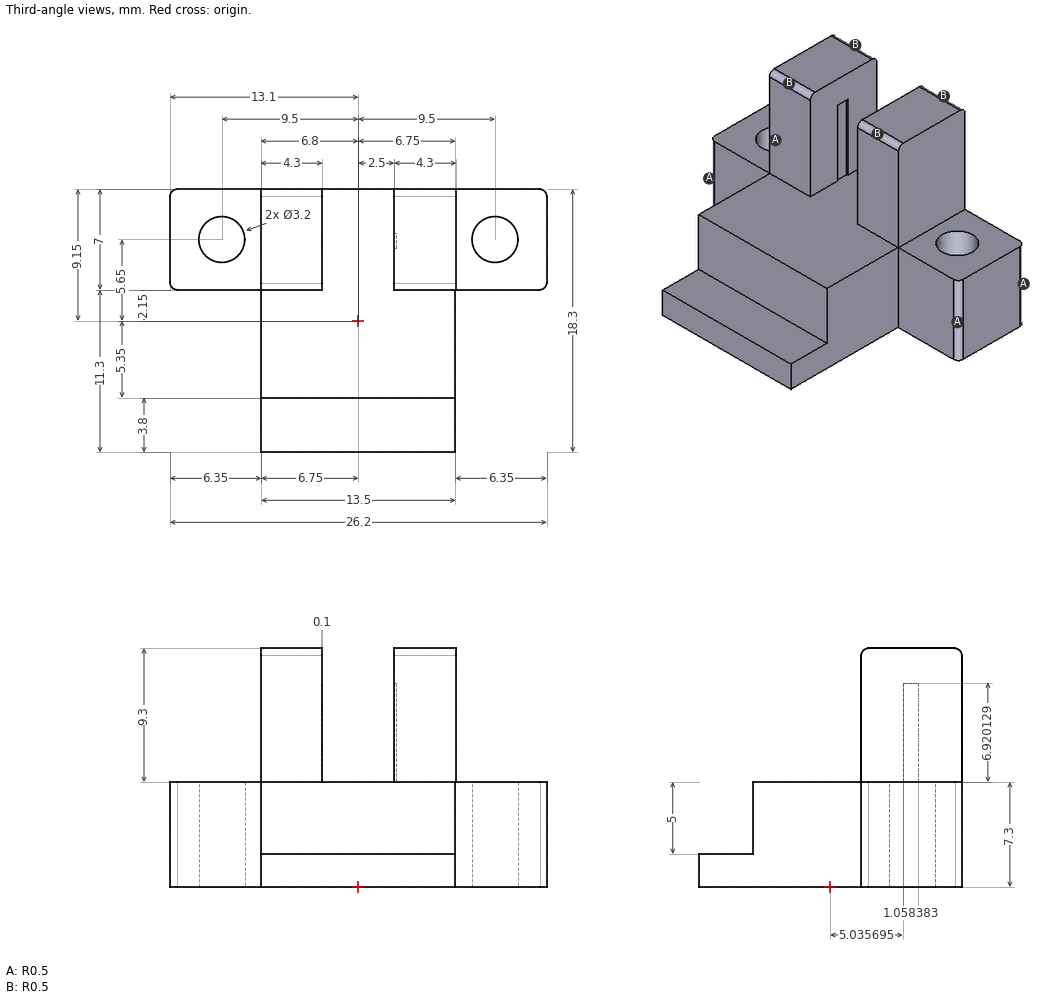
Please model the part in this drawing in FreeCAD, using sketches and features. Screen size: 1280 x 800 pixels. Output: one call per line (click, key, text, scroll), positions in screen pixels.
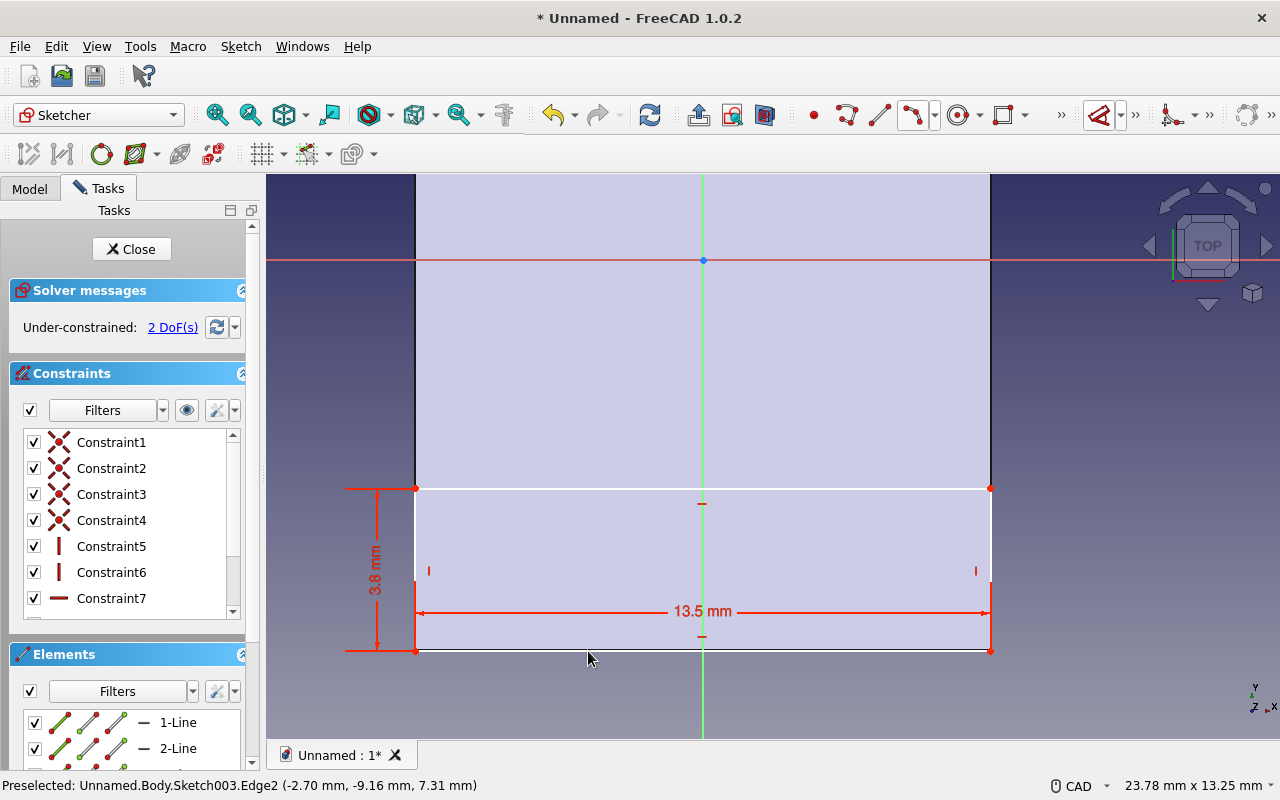
click(415, 489)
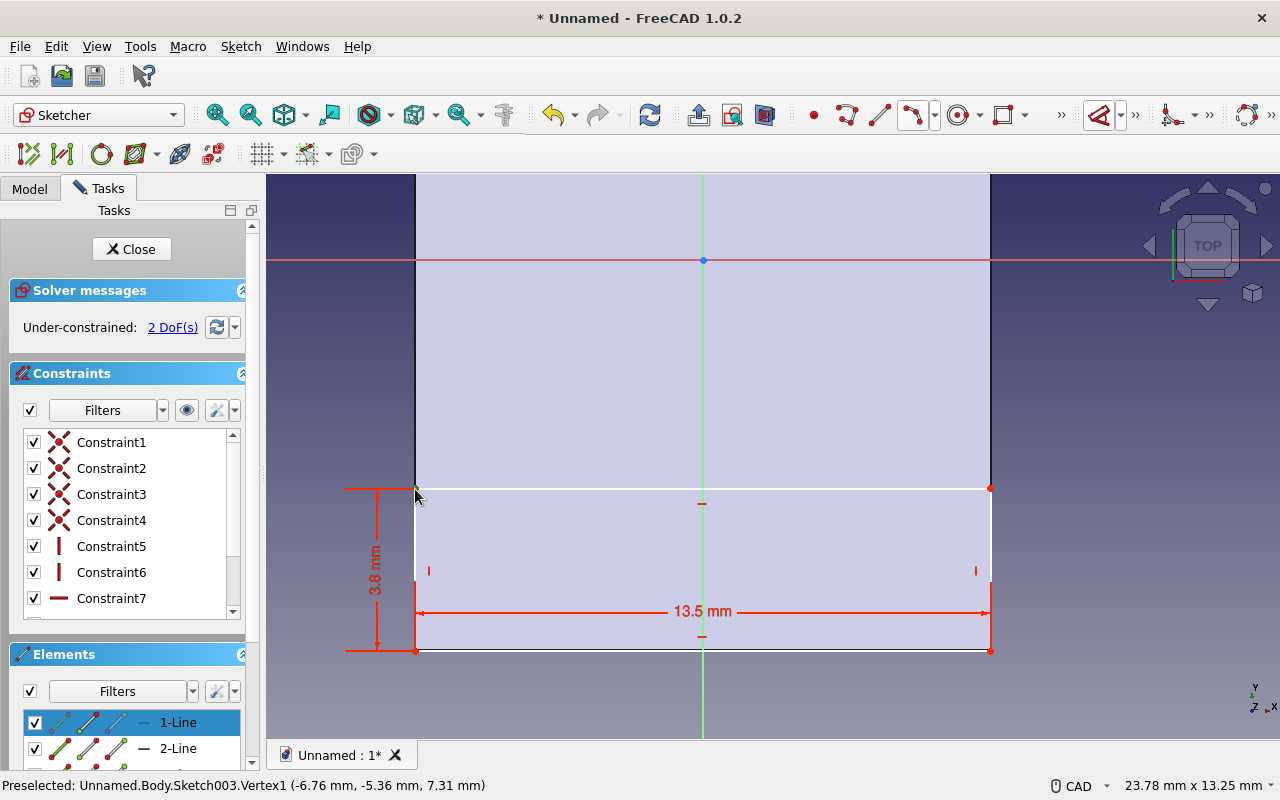
key(l)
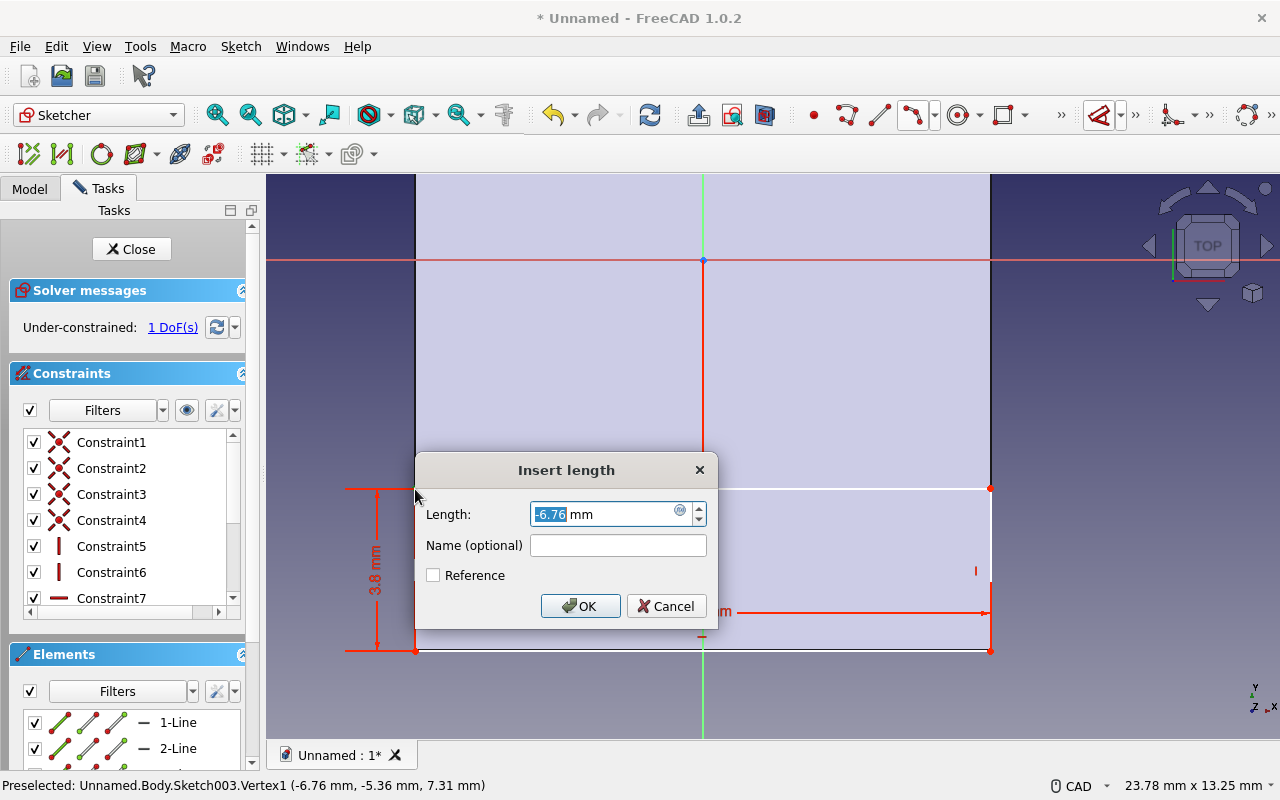
text(-6.75)
key(Return)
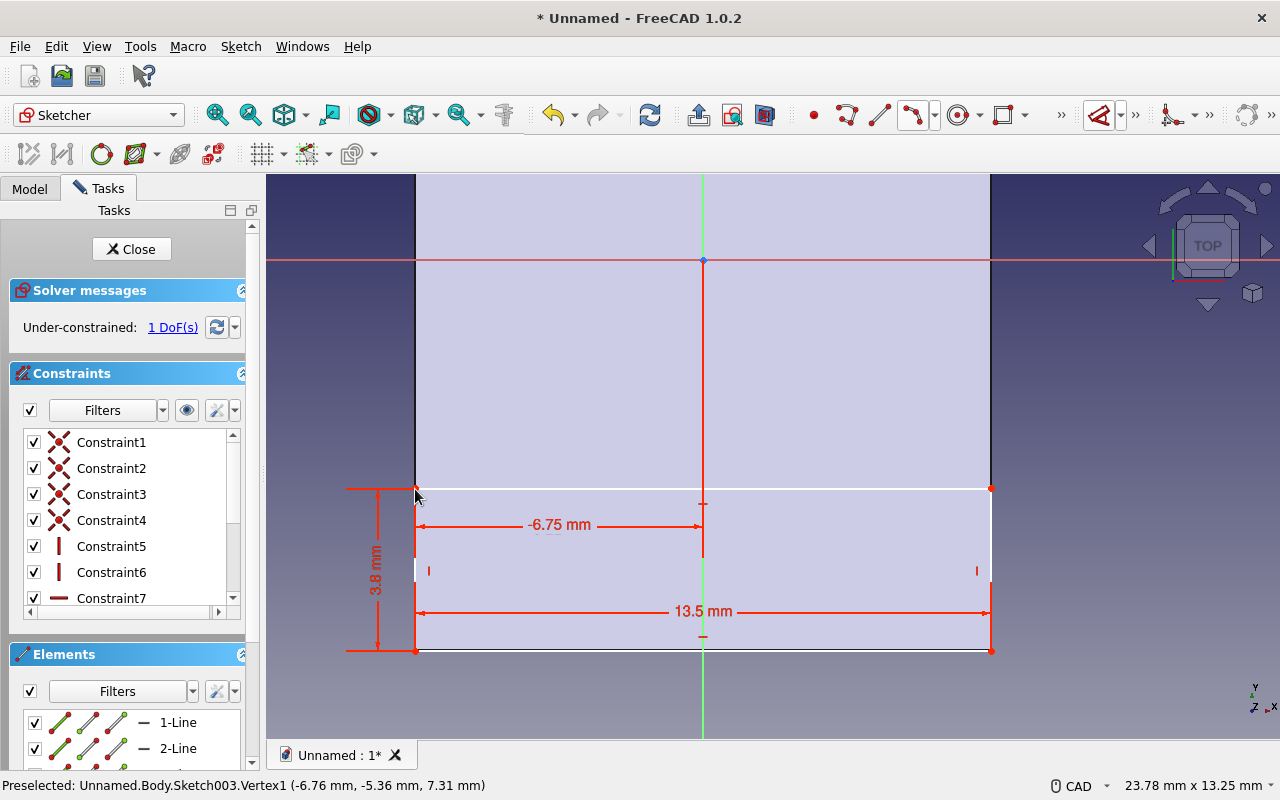
click(415, 489)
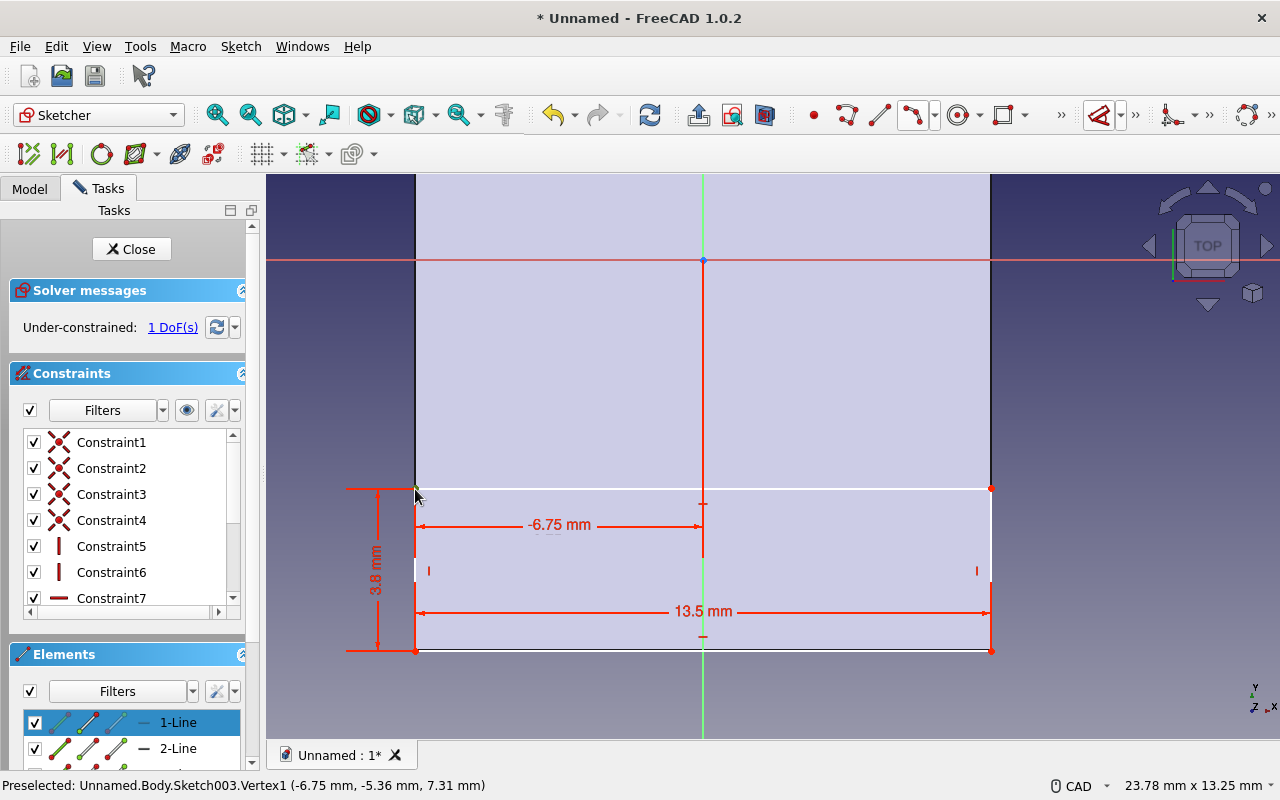
key(i)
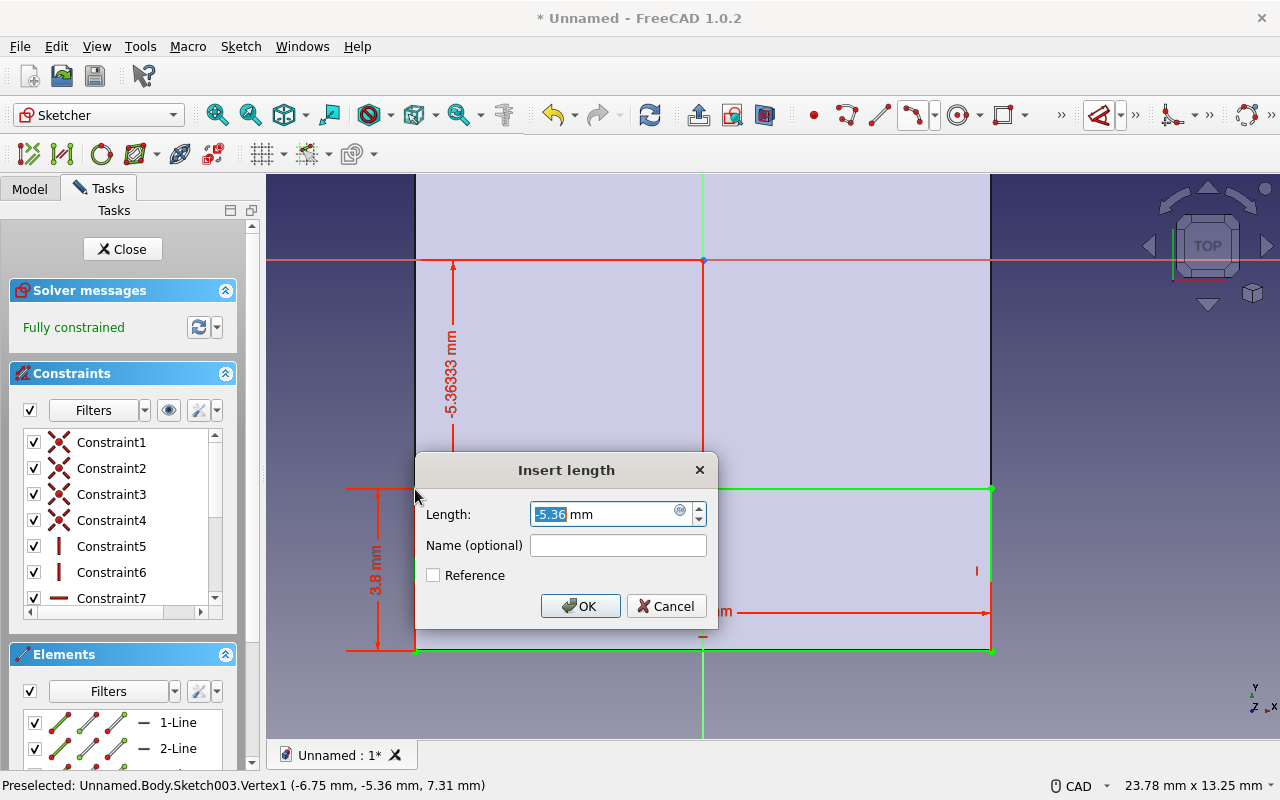
text(-5.35)
key(Return)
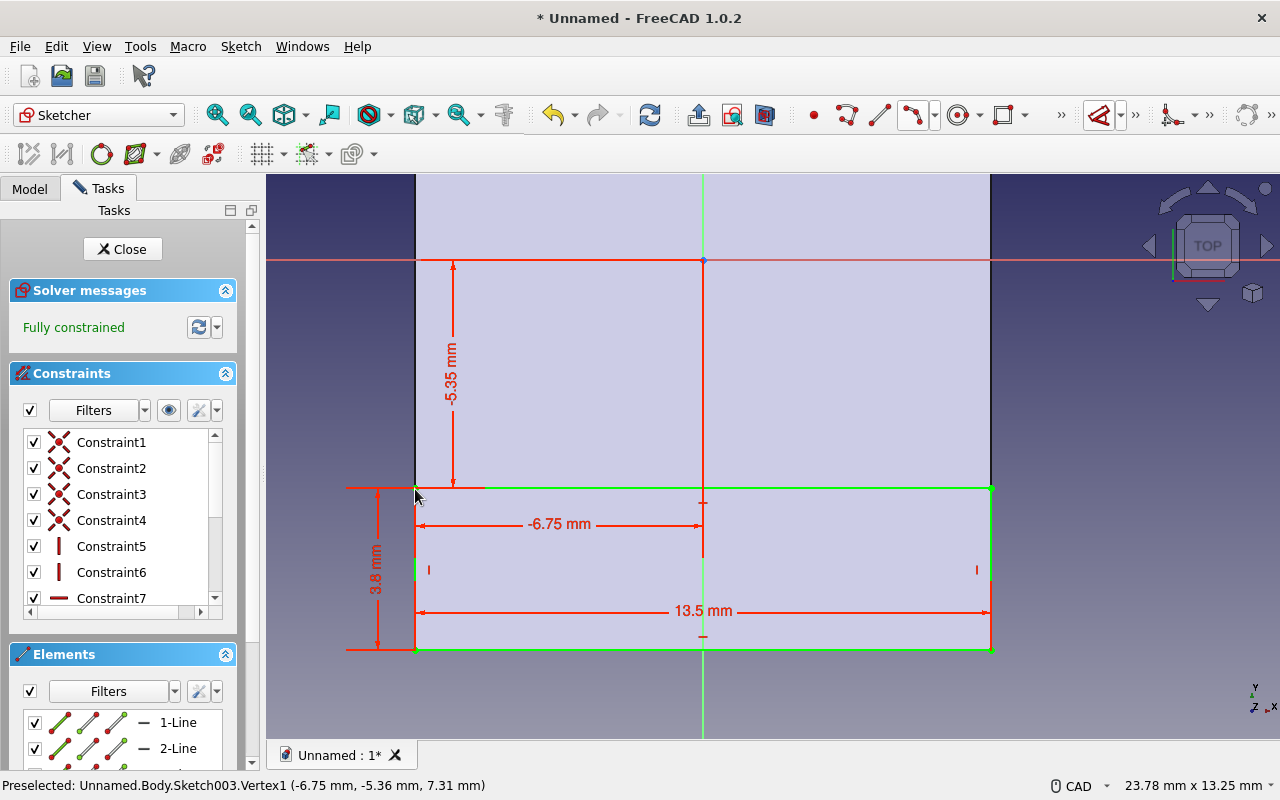
click(123, 249)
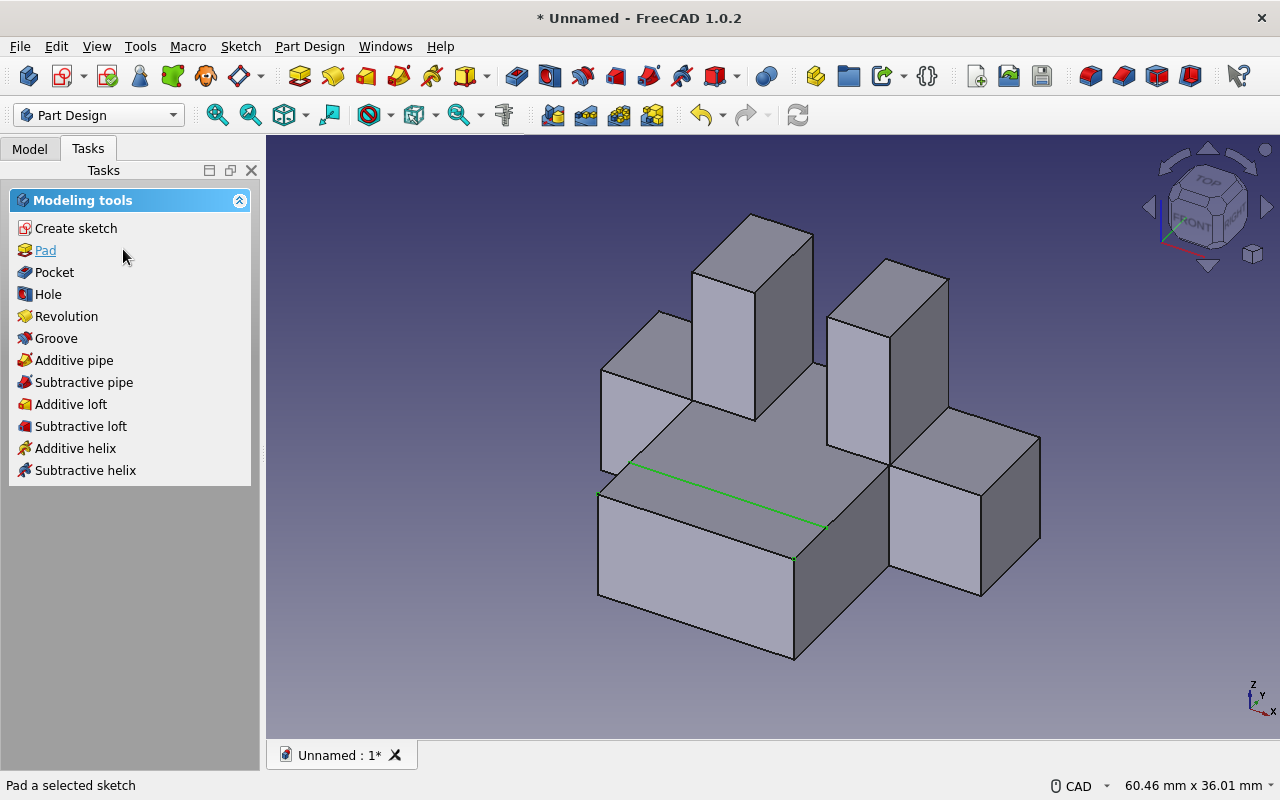
click(517, 76)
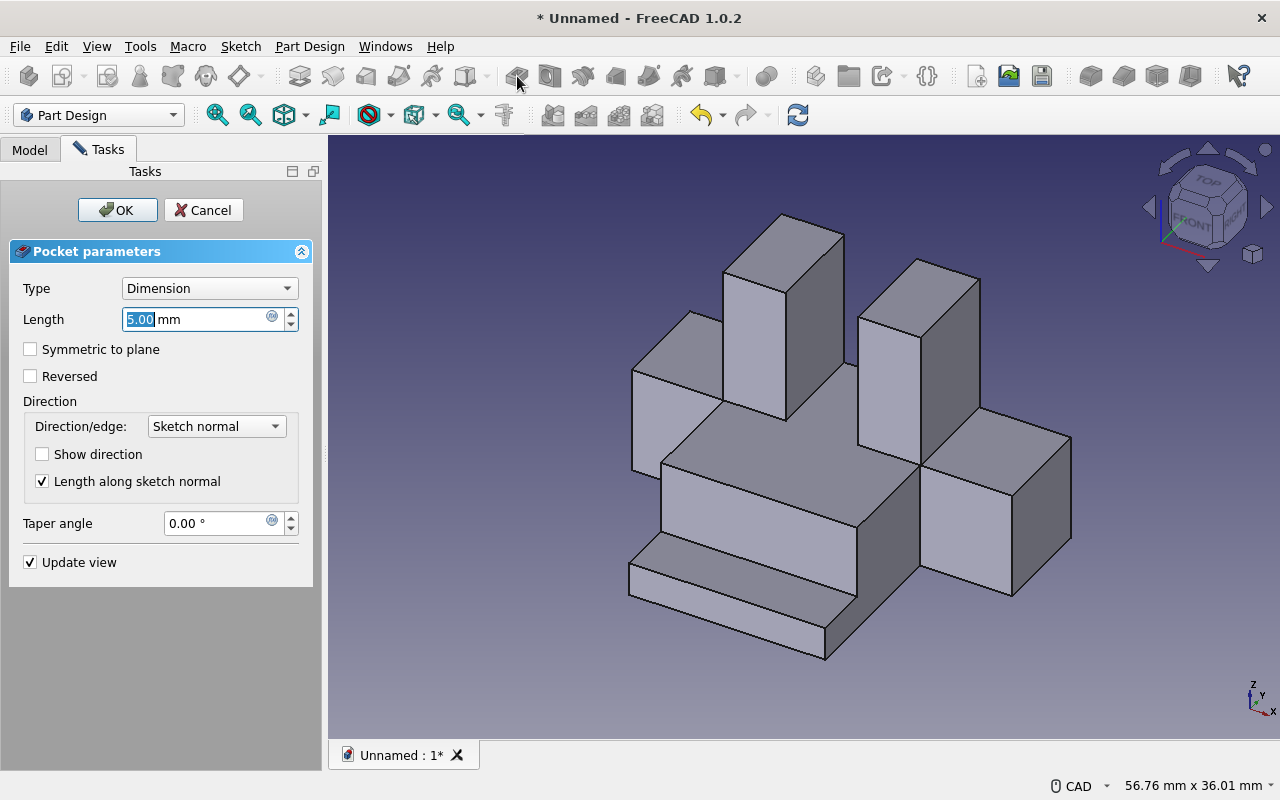
text(5)
key(Tab)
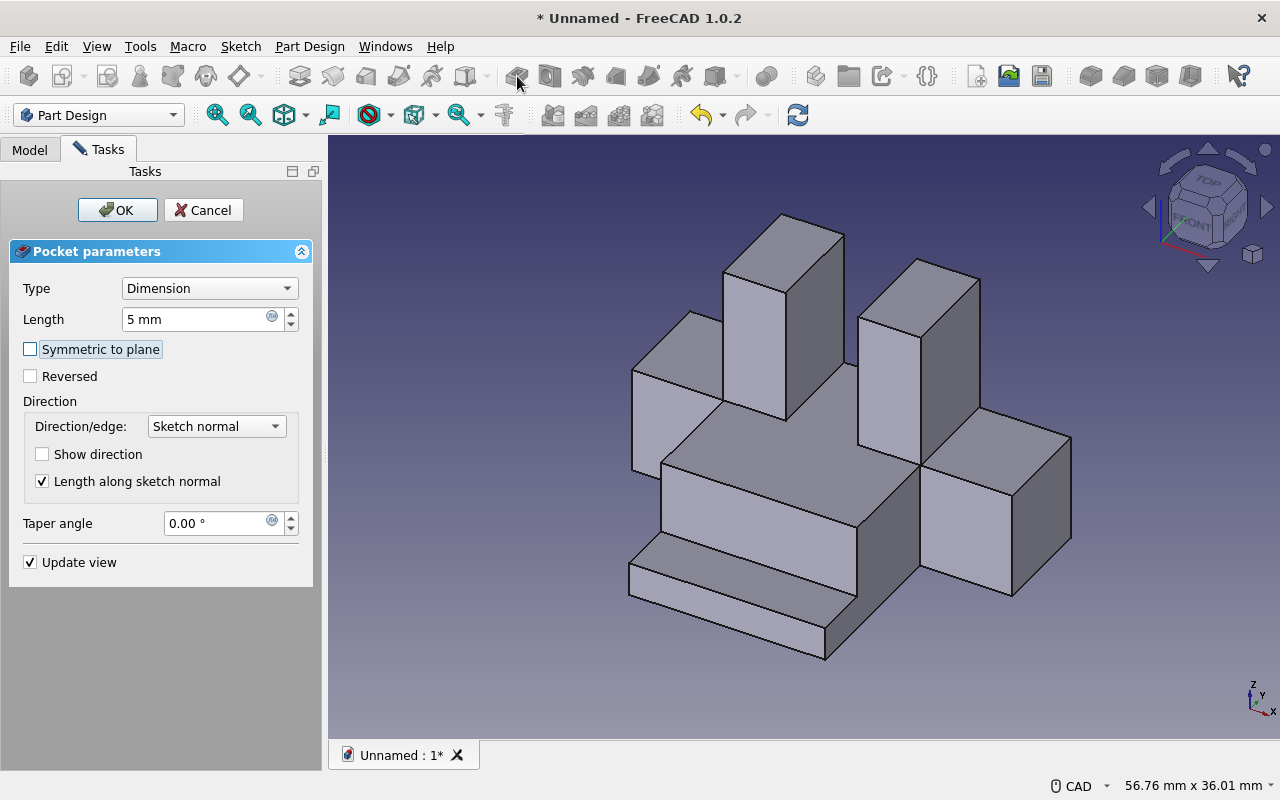
click(118, 210)